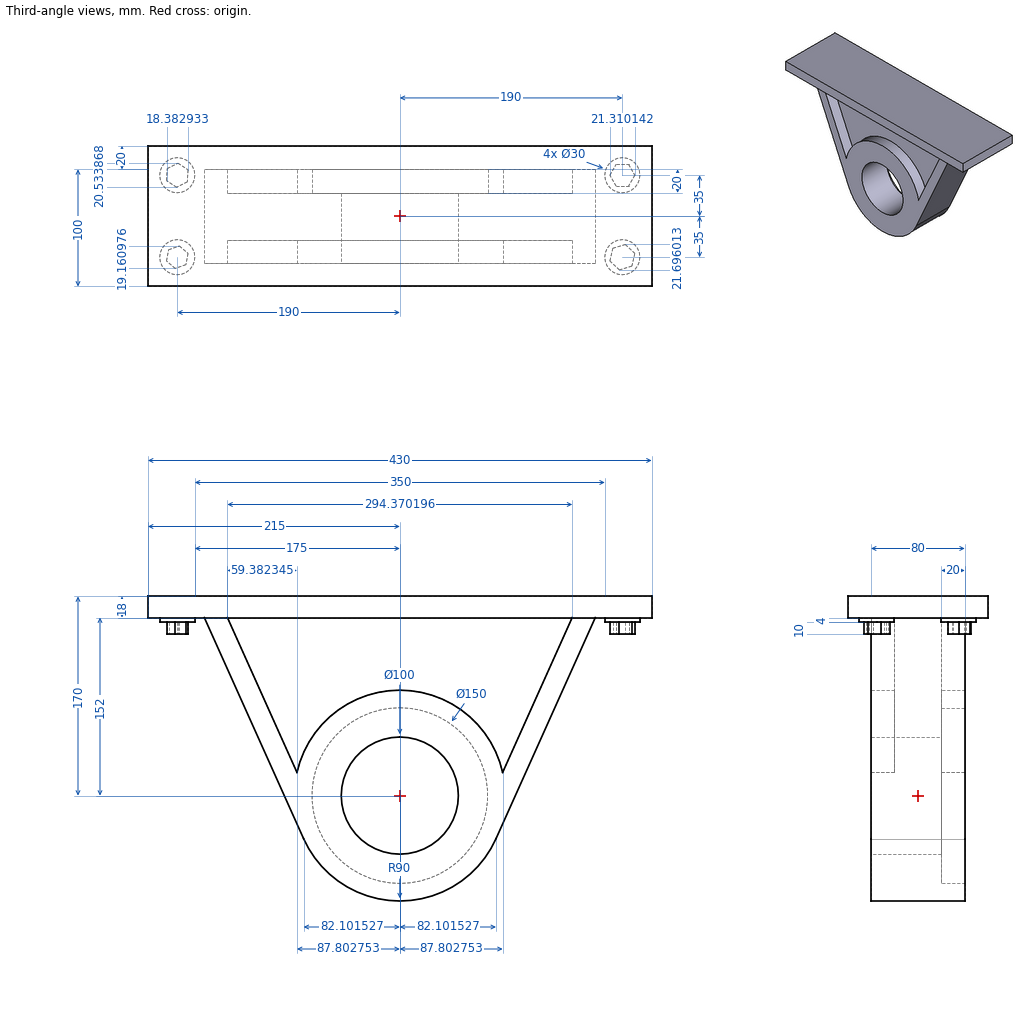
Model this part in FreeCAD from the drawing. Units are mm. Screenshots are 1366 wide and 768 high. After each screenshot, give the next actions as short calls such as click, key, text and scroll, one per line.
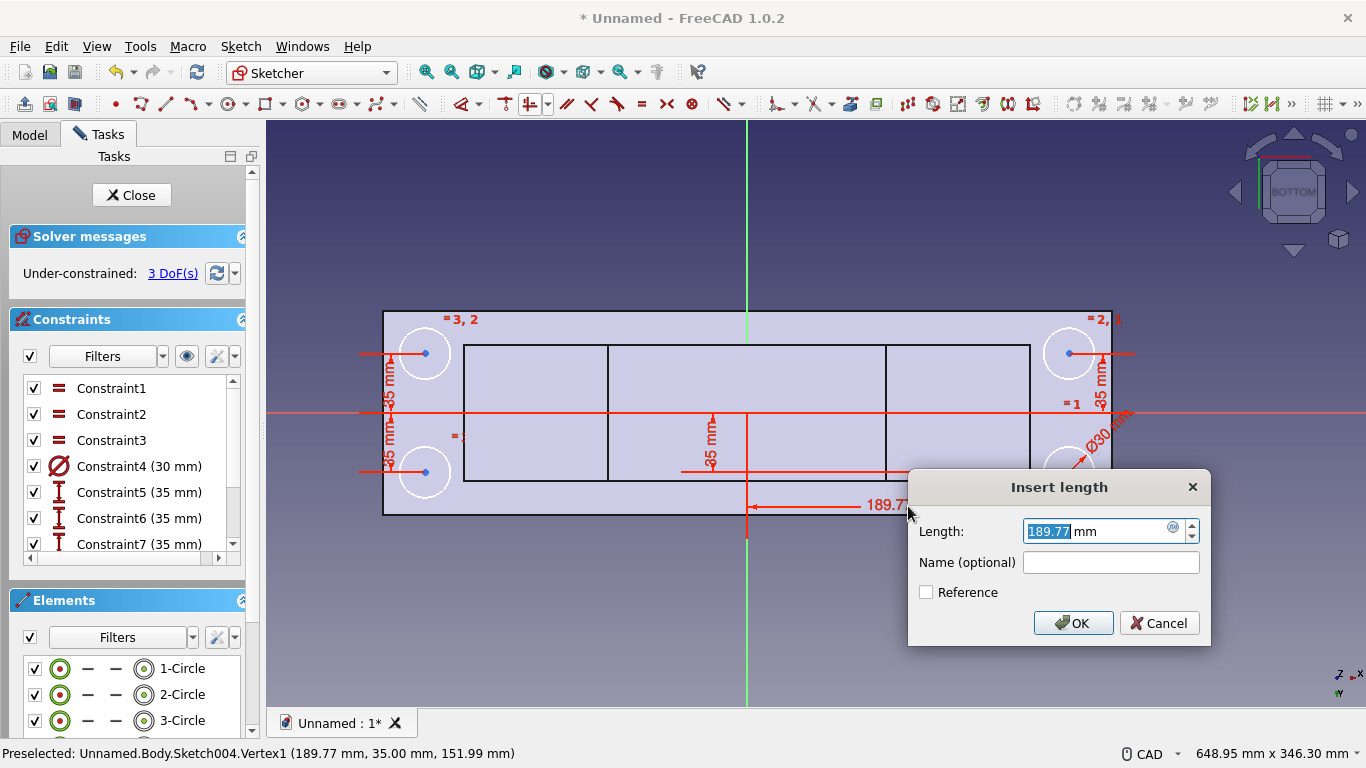
text(190)
key(Return)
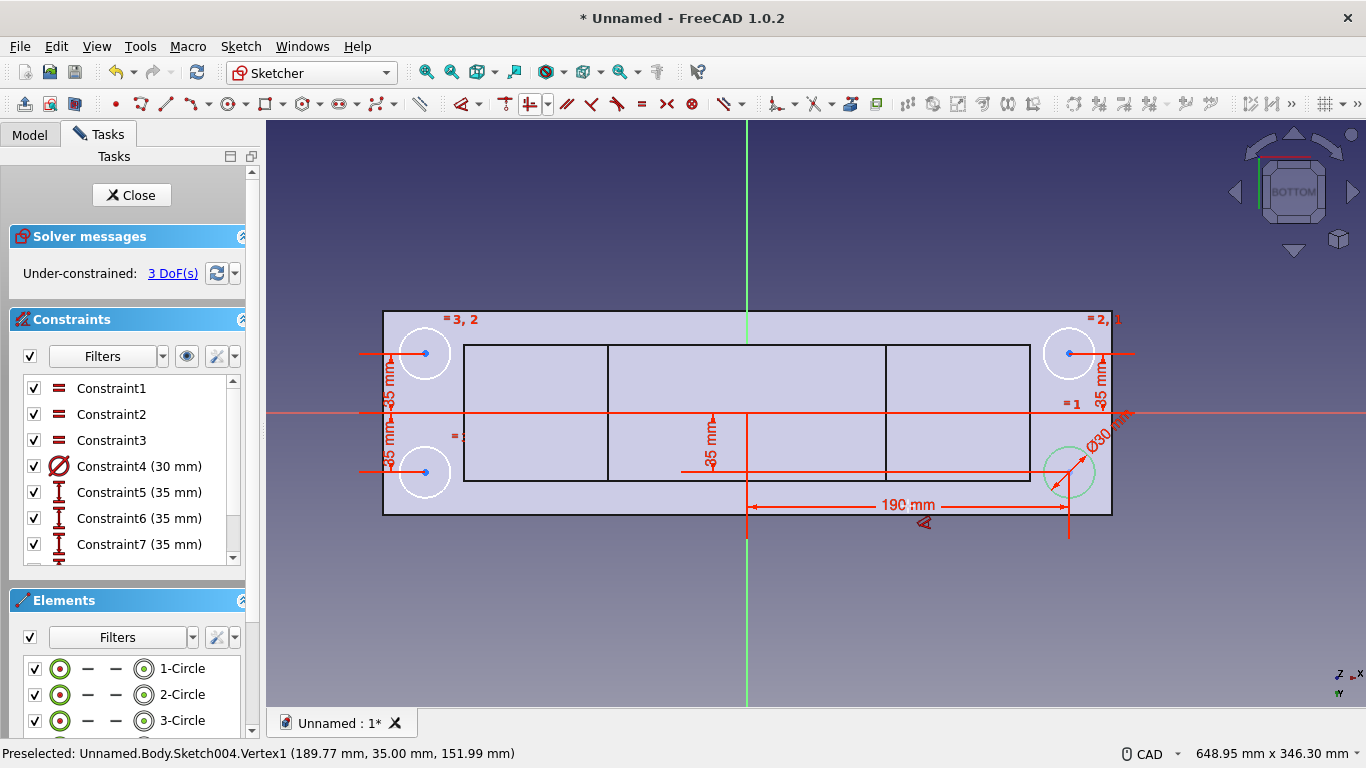
click(1069, 354)
click(908, 320)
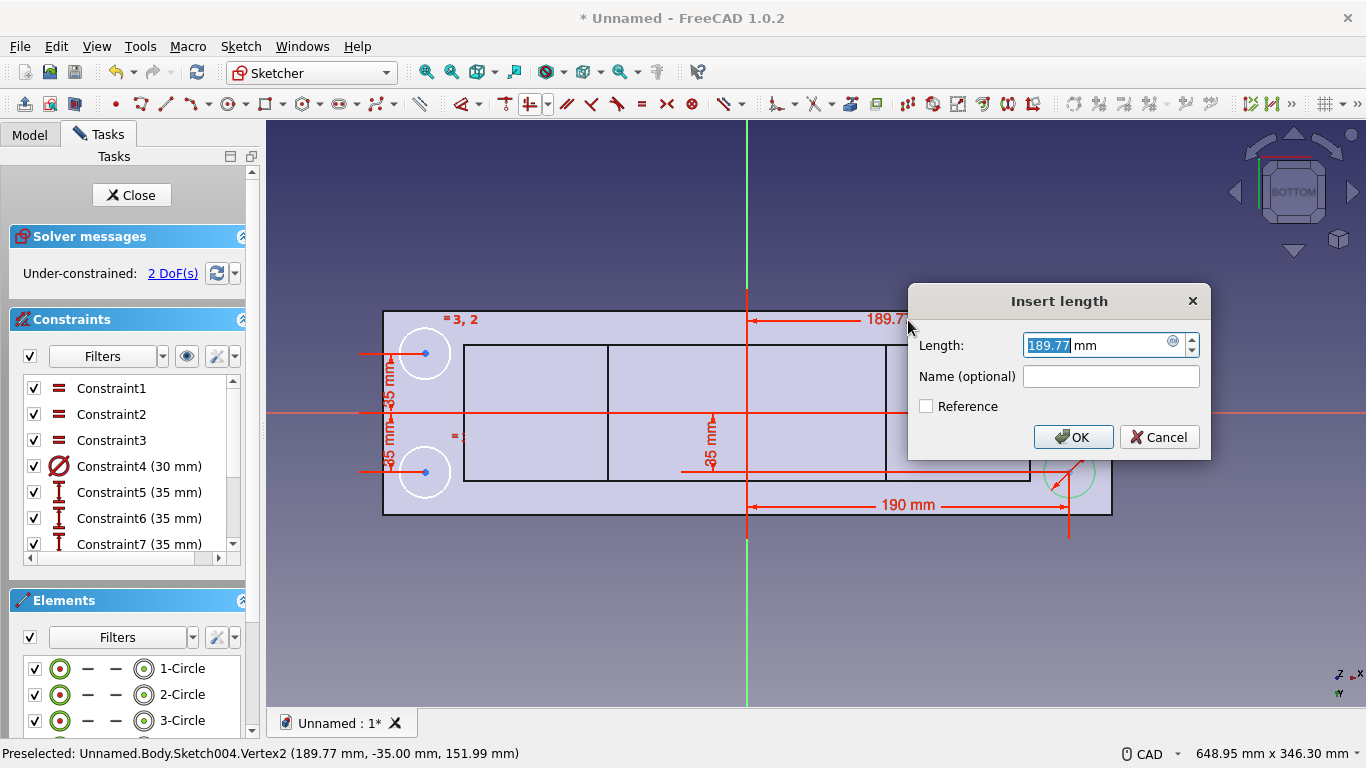
text(190)
key(Return)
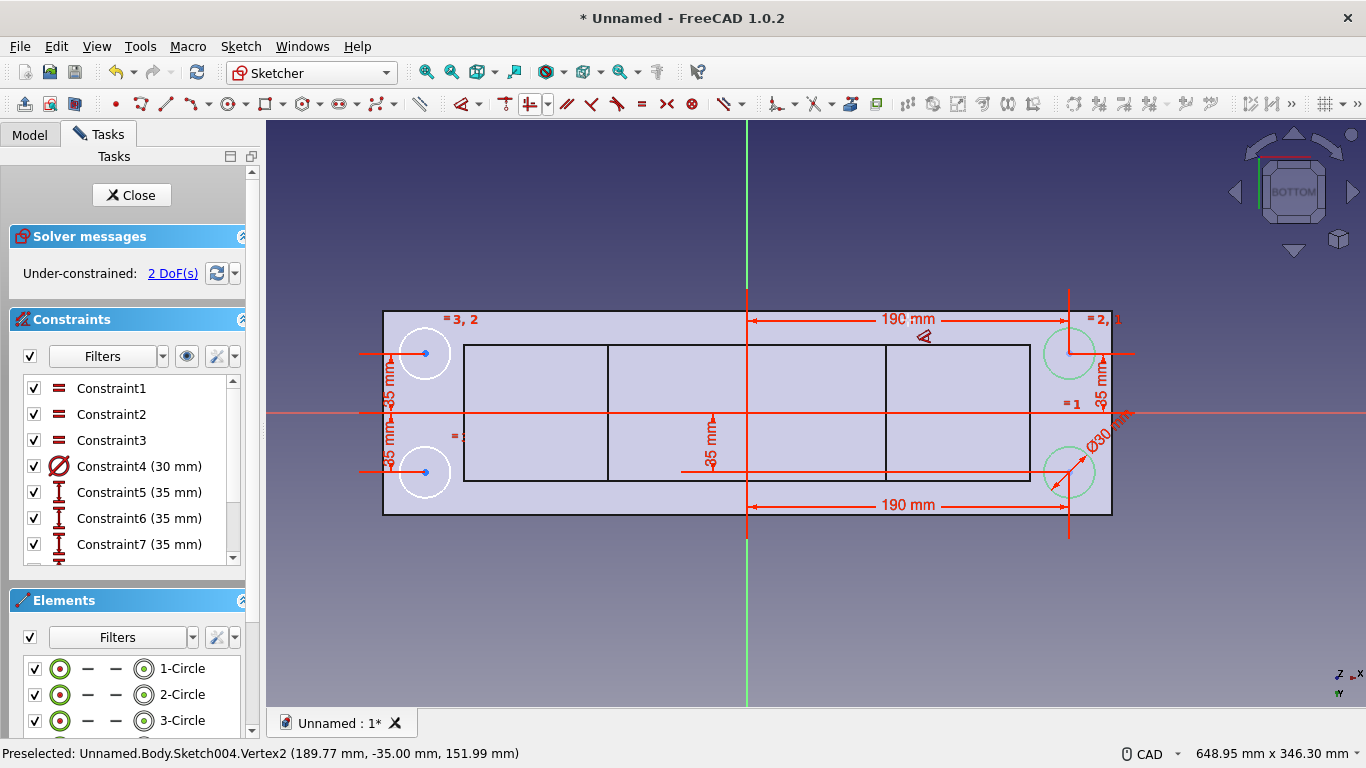
click(425, 354)
click(586, 320)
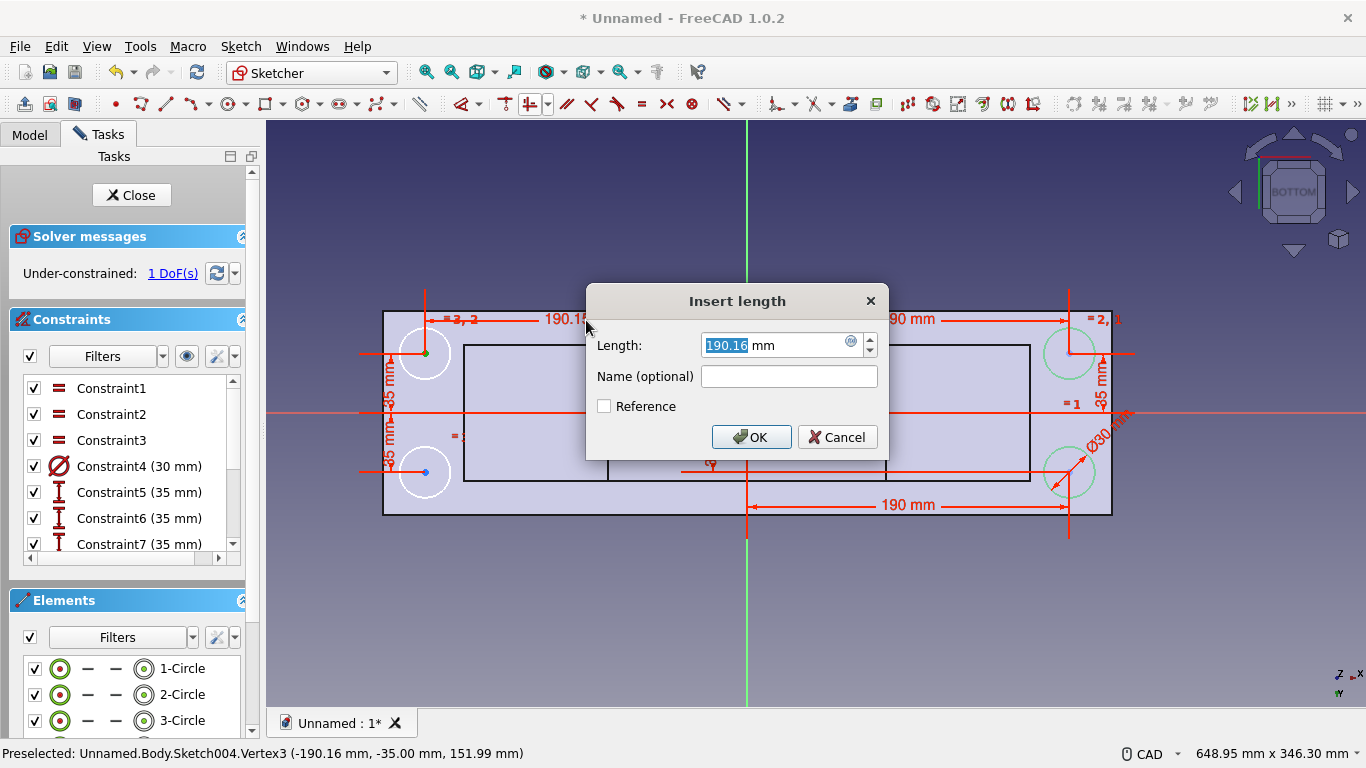
text(190)
key(Return)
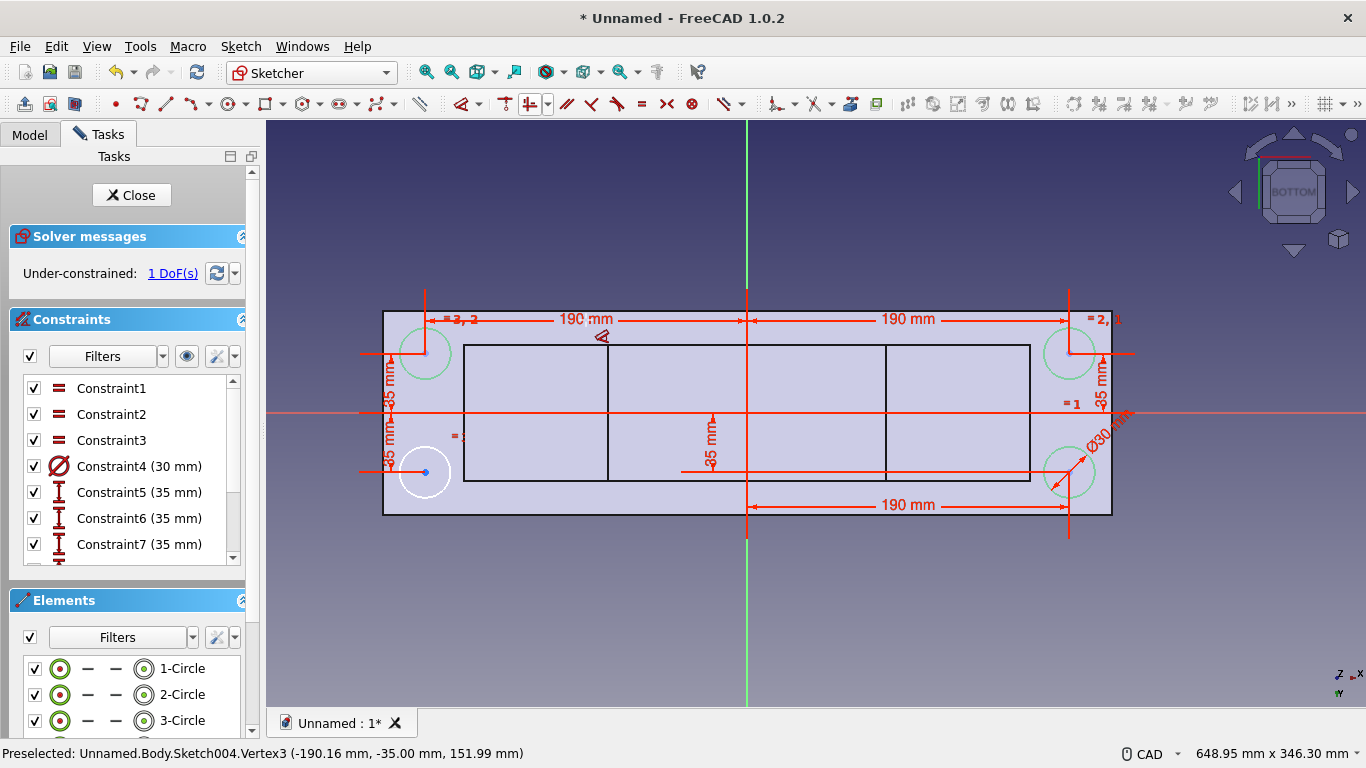
click(425, 472)
click(586, 506)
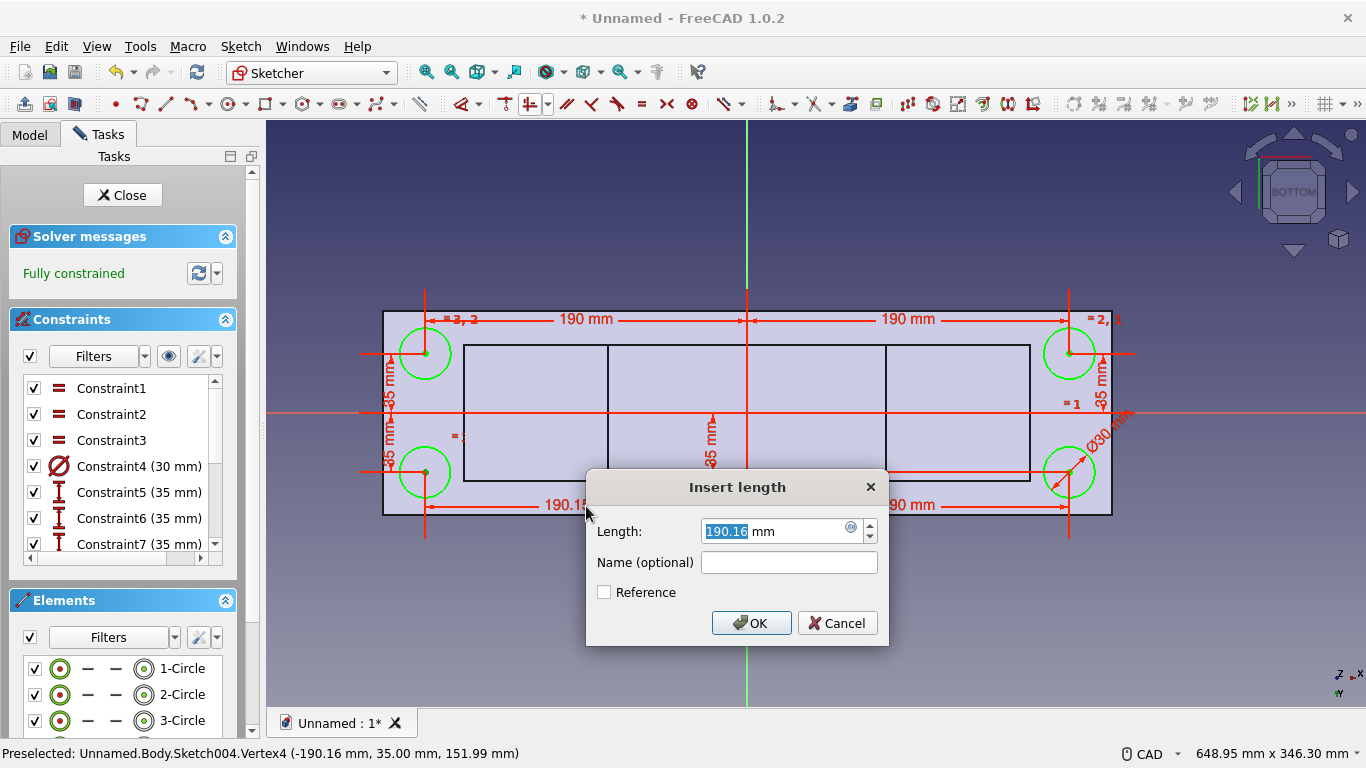
text(190)
key(Return)
key(Escape)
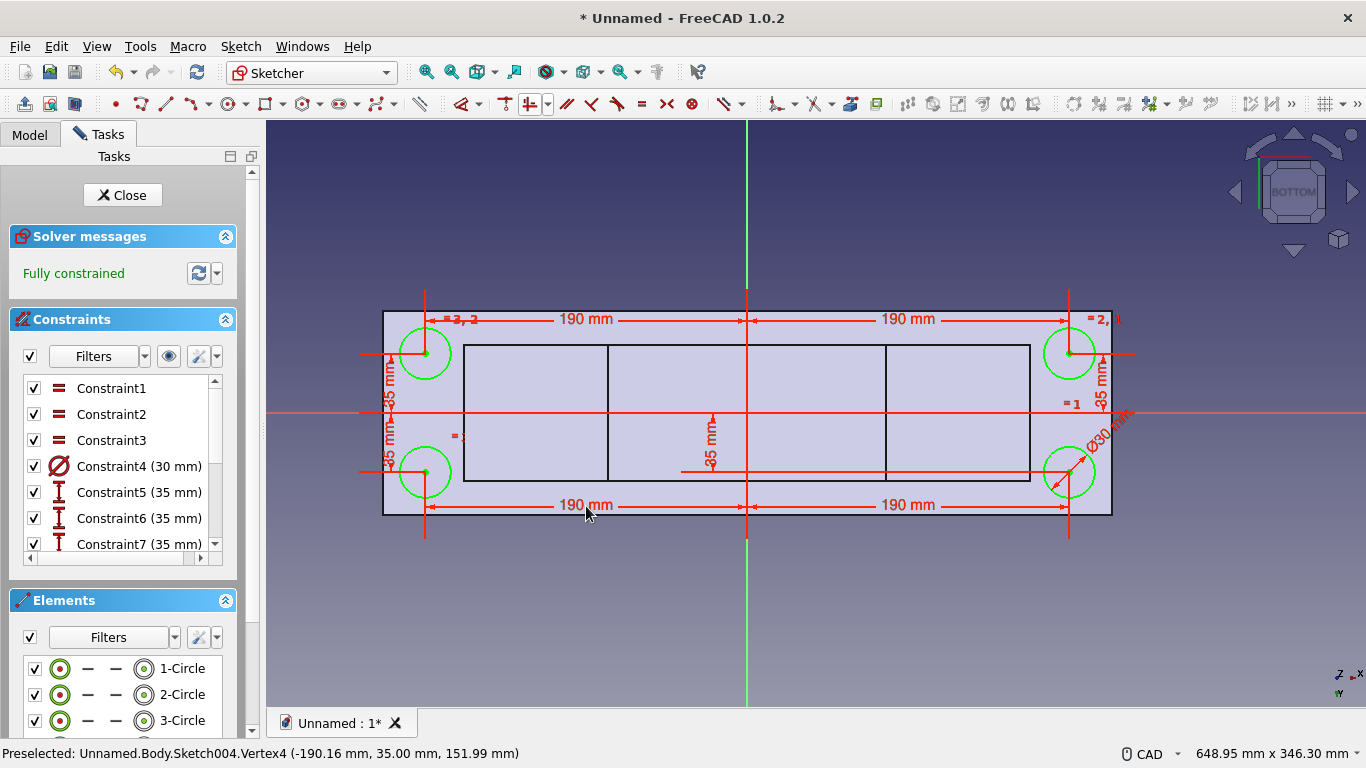
click(123, 195)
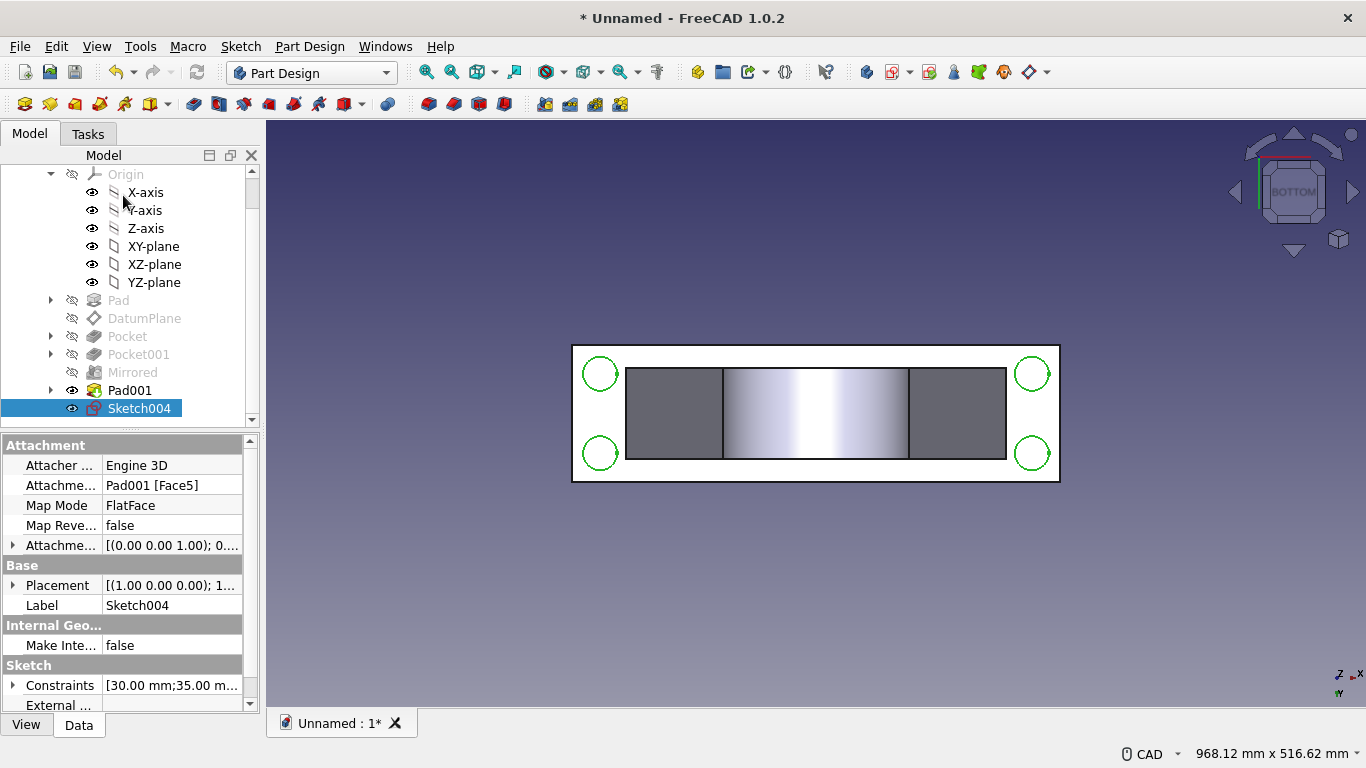
click(25, 104)